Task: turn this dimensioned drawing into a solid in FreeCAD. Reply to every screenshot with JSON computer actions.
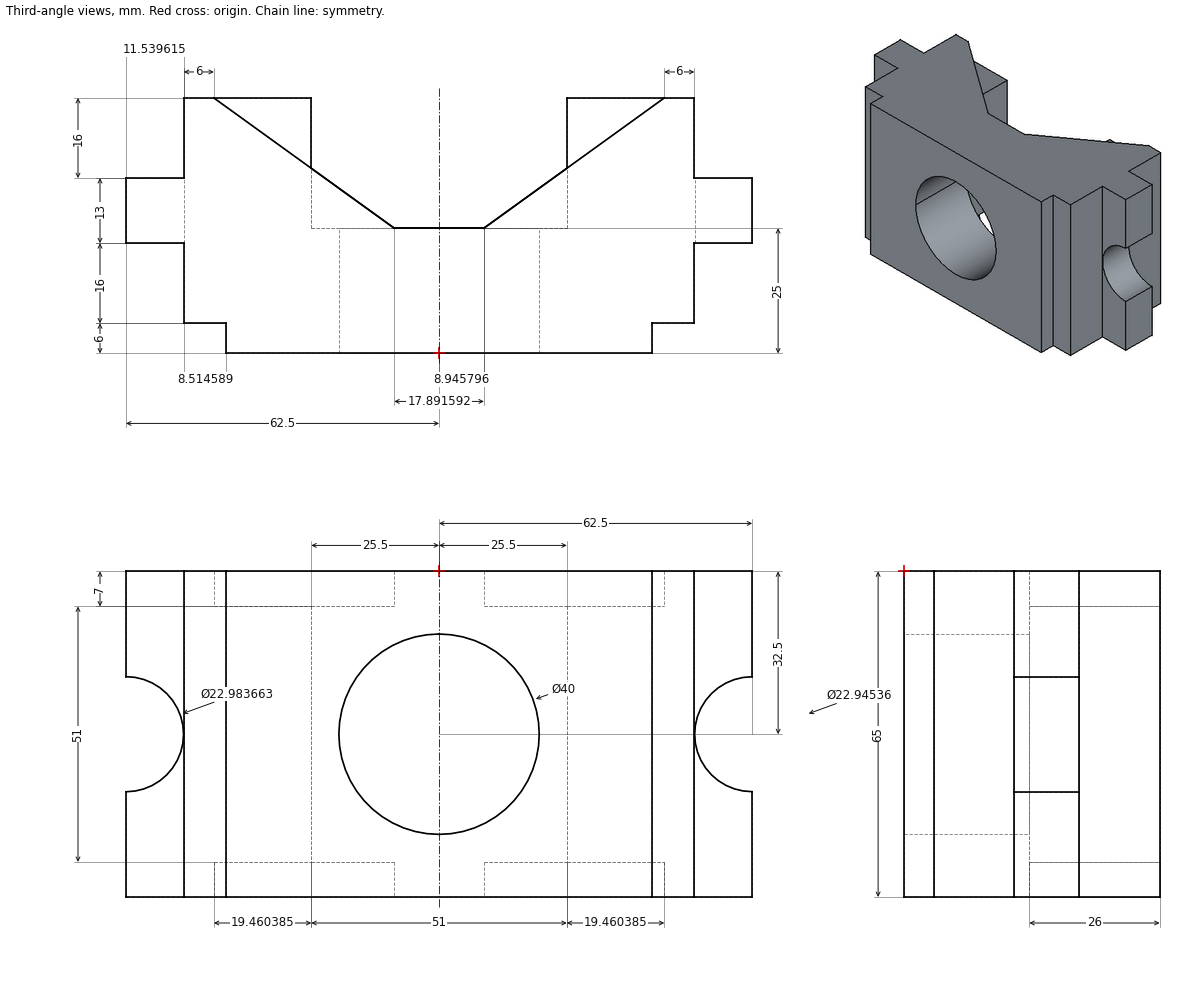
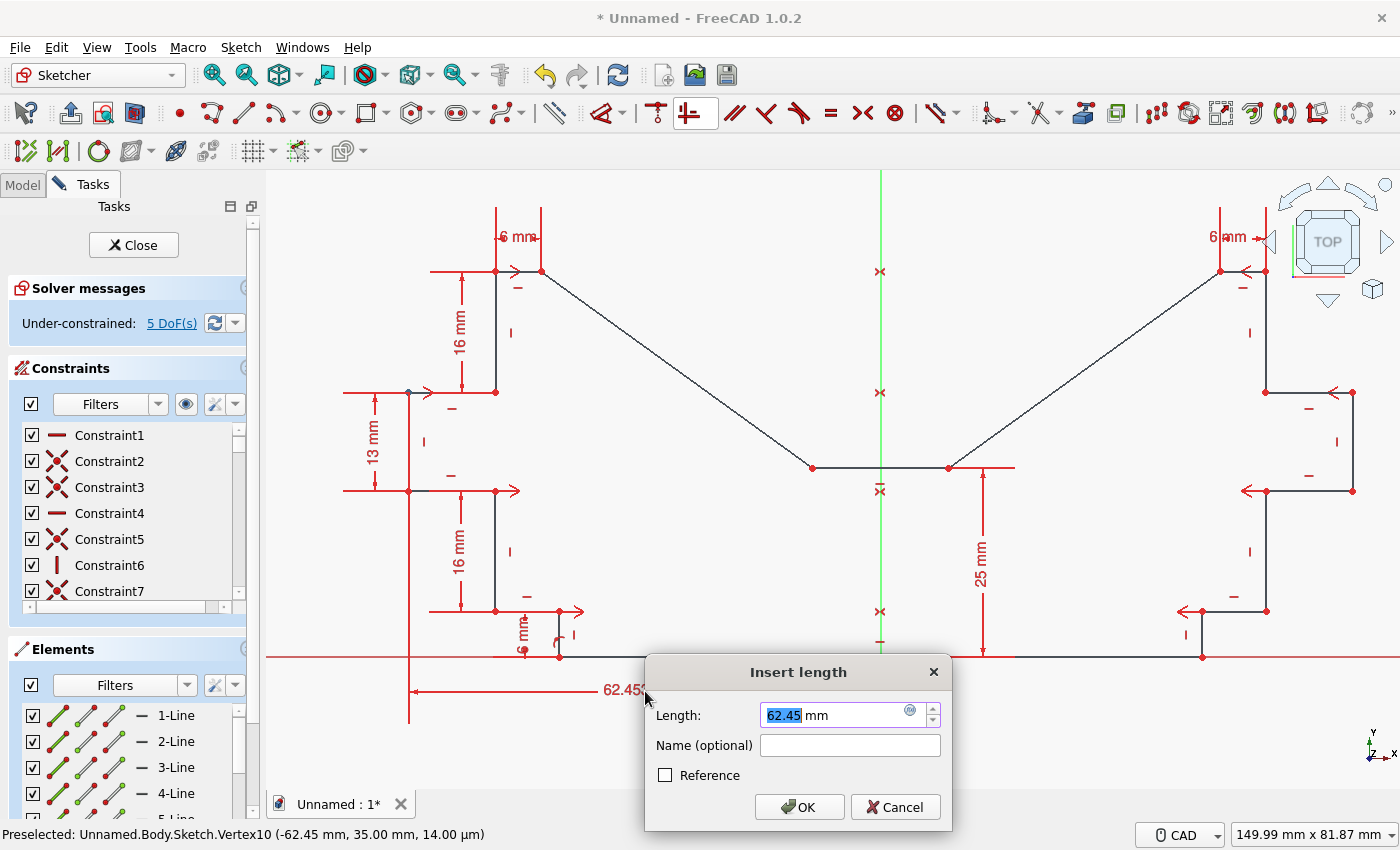
{"action": "type", "text": "62.5"}
{"action": "key", "text": "Return"}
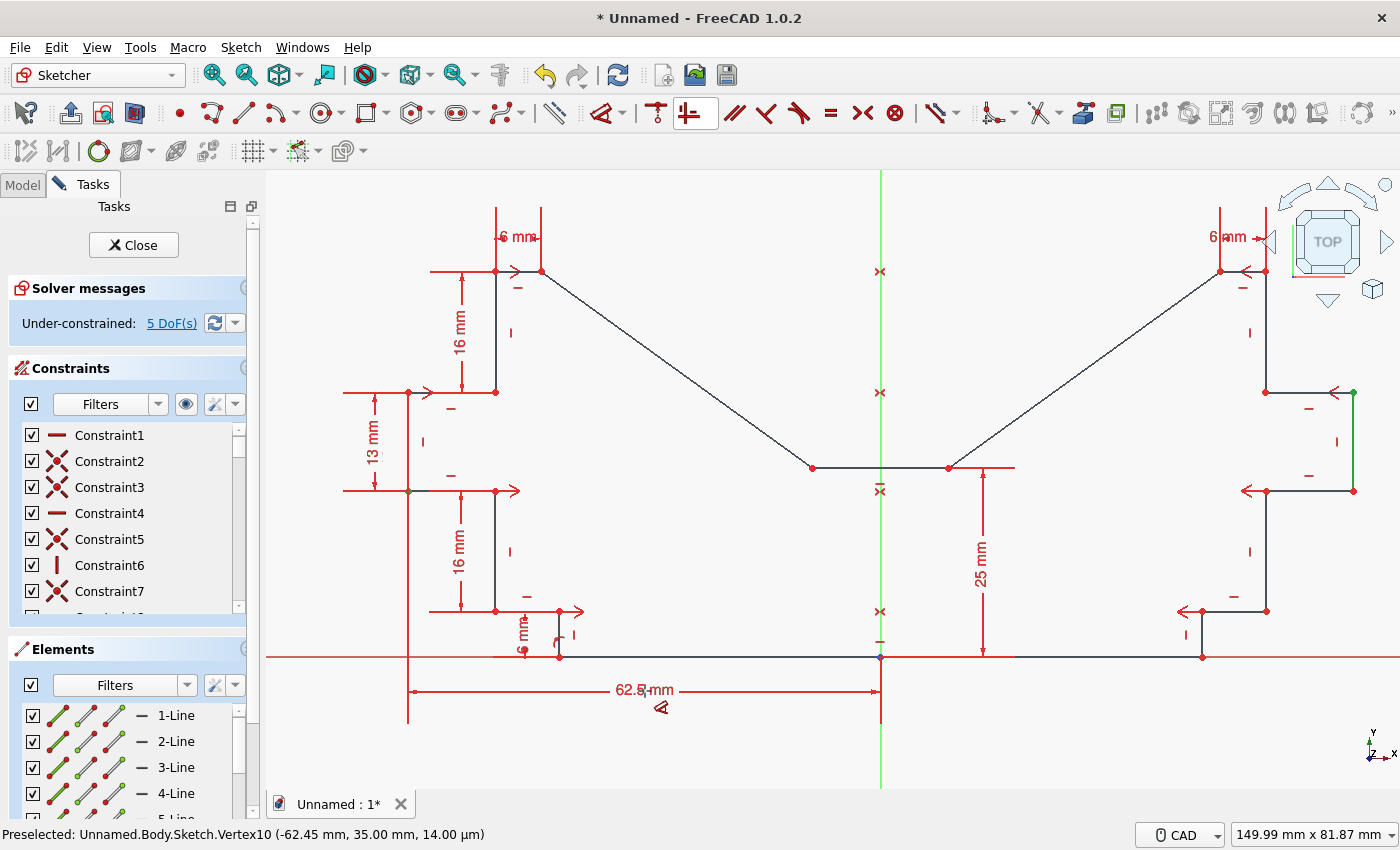
{"action": "left_click", "coordinate": [514, 612]}
{"action": "left_click", "coordinate": [527, 578]}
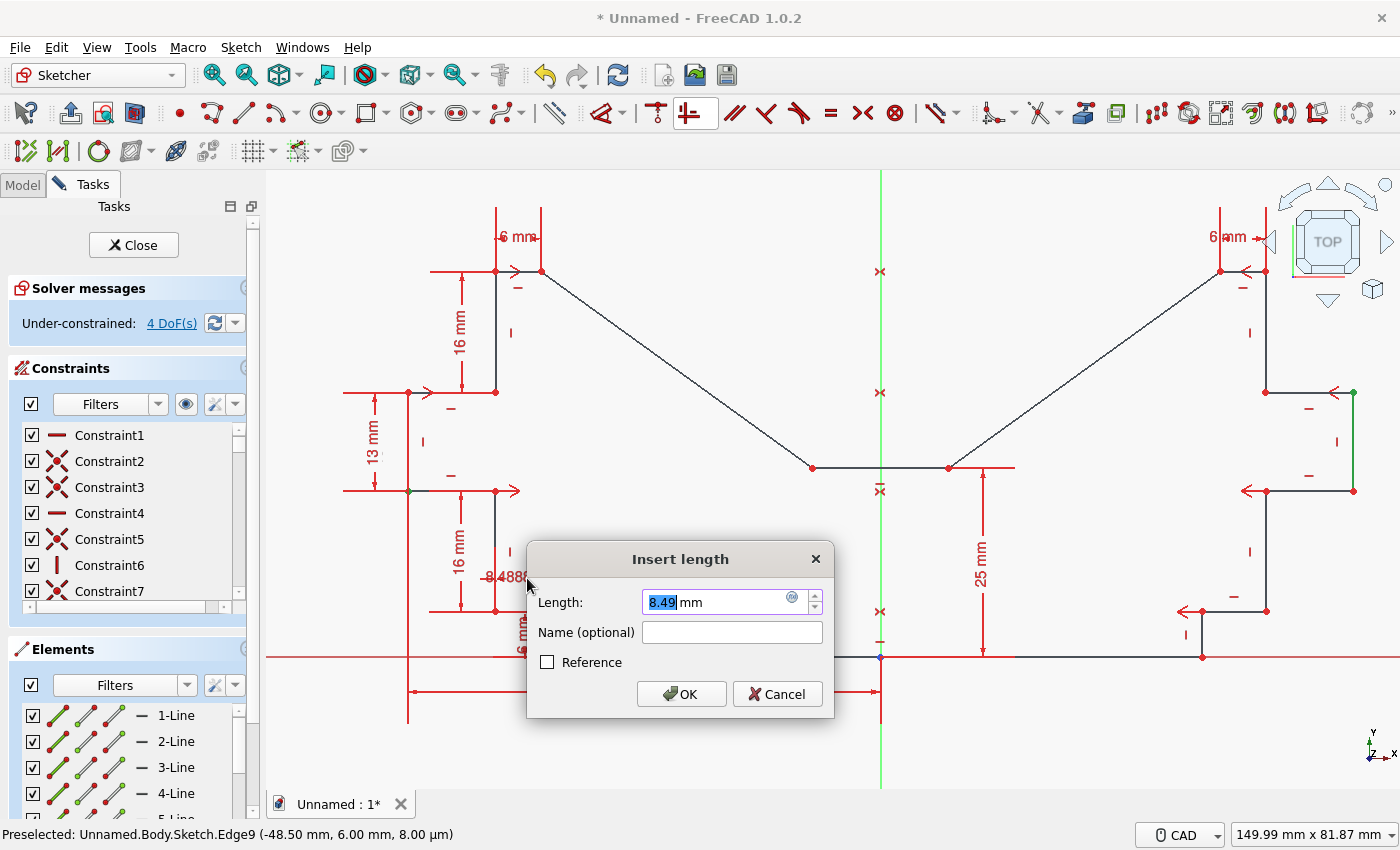
{"action": "type", "text": "8.514589"}
{"action": "key", "text": "Return"}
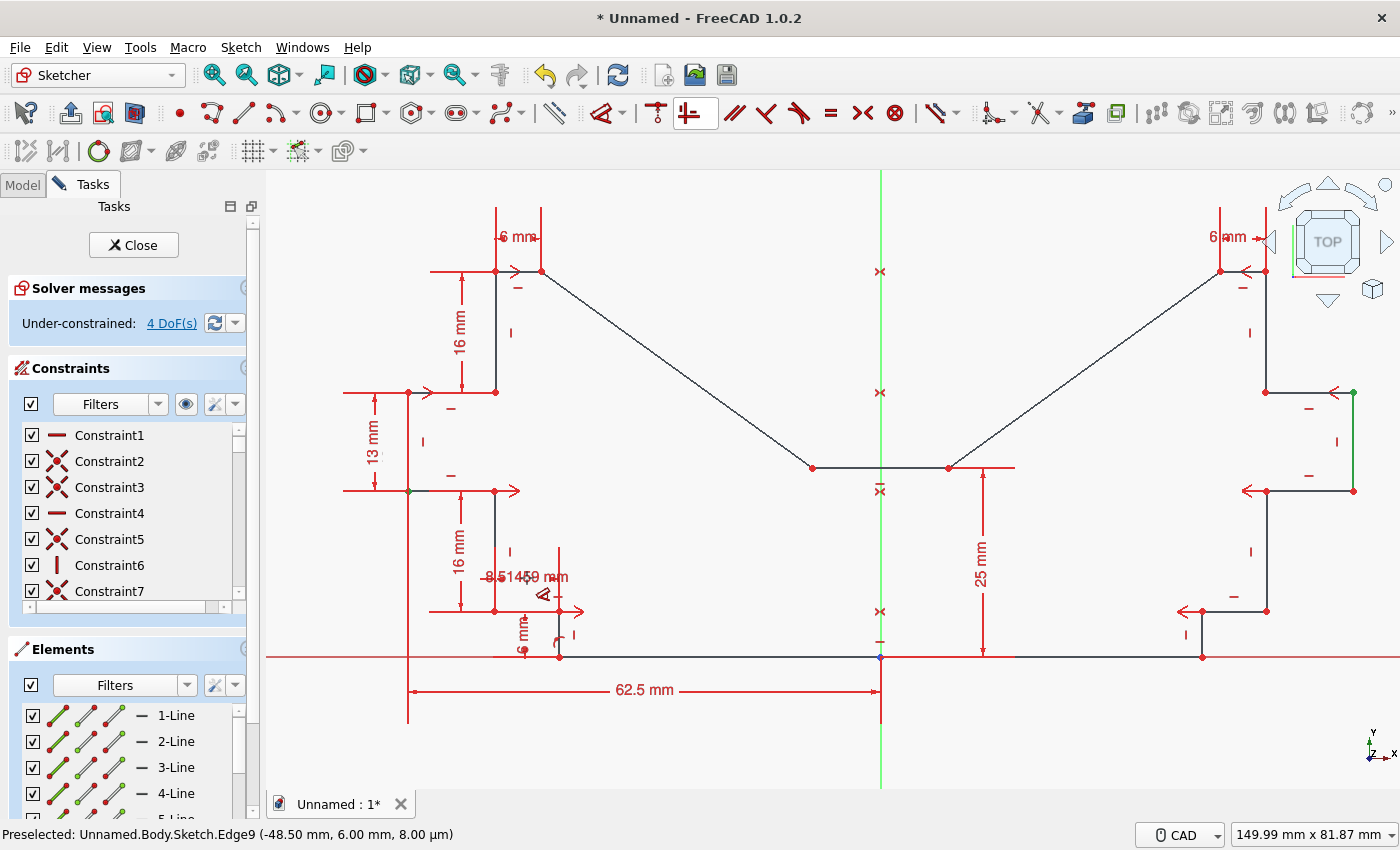
{"action": "left_click", "coordinate": [908, 468]}
{"action": "left_click", "coordinate": [849, 502]}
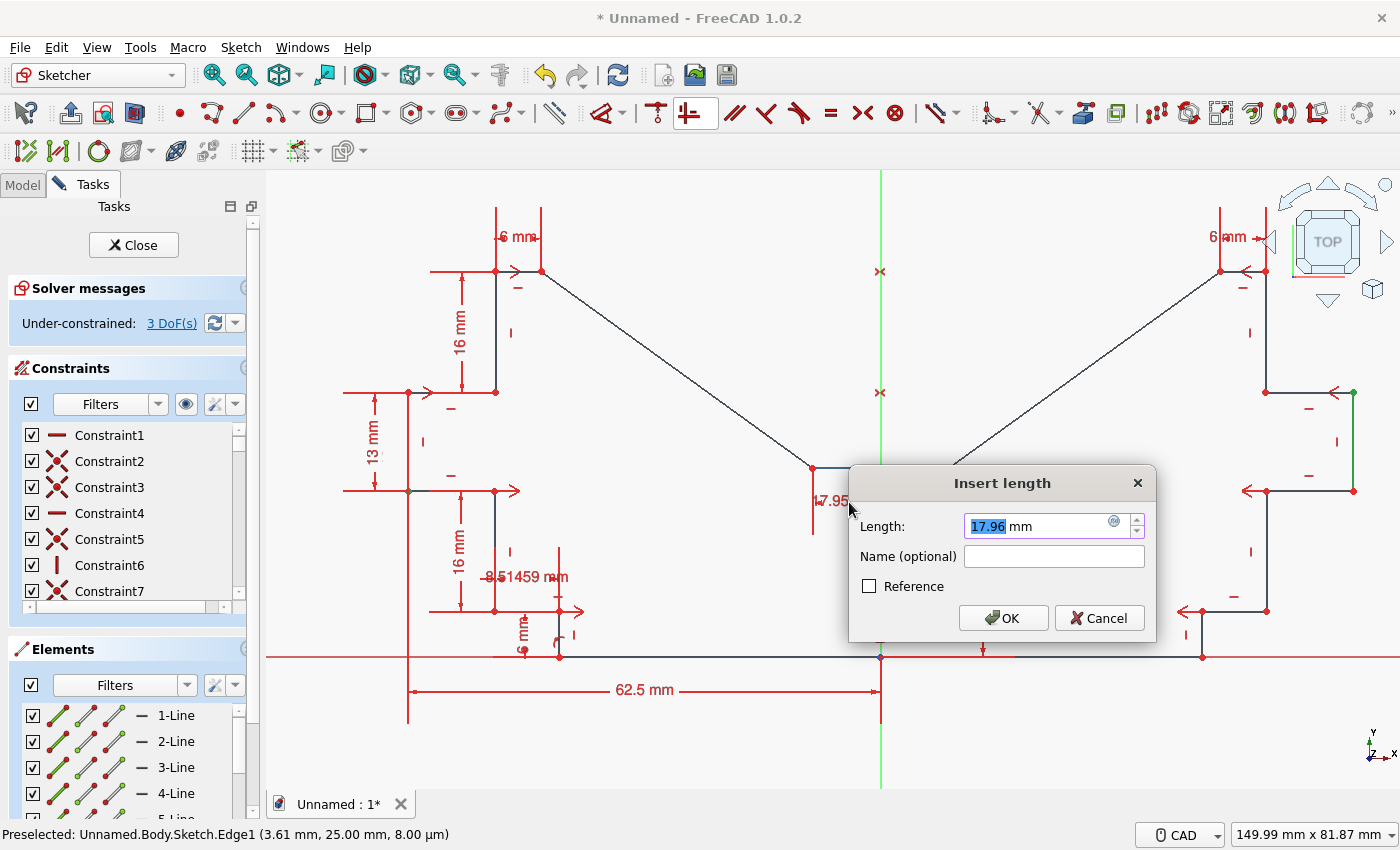
{"action": "type", "text": "17.891592"}
{"action": "key", "text": "Return"}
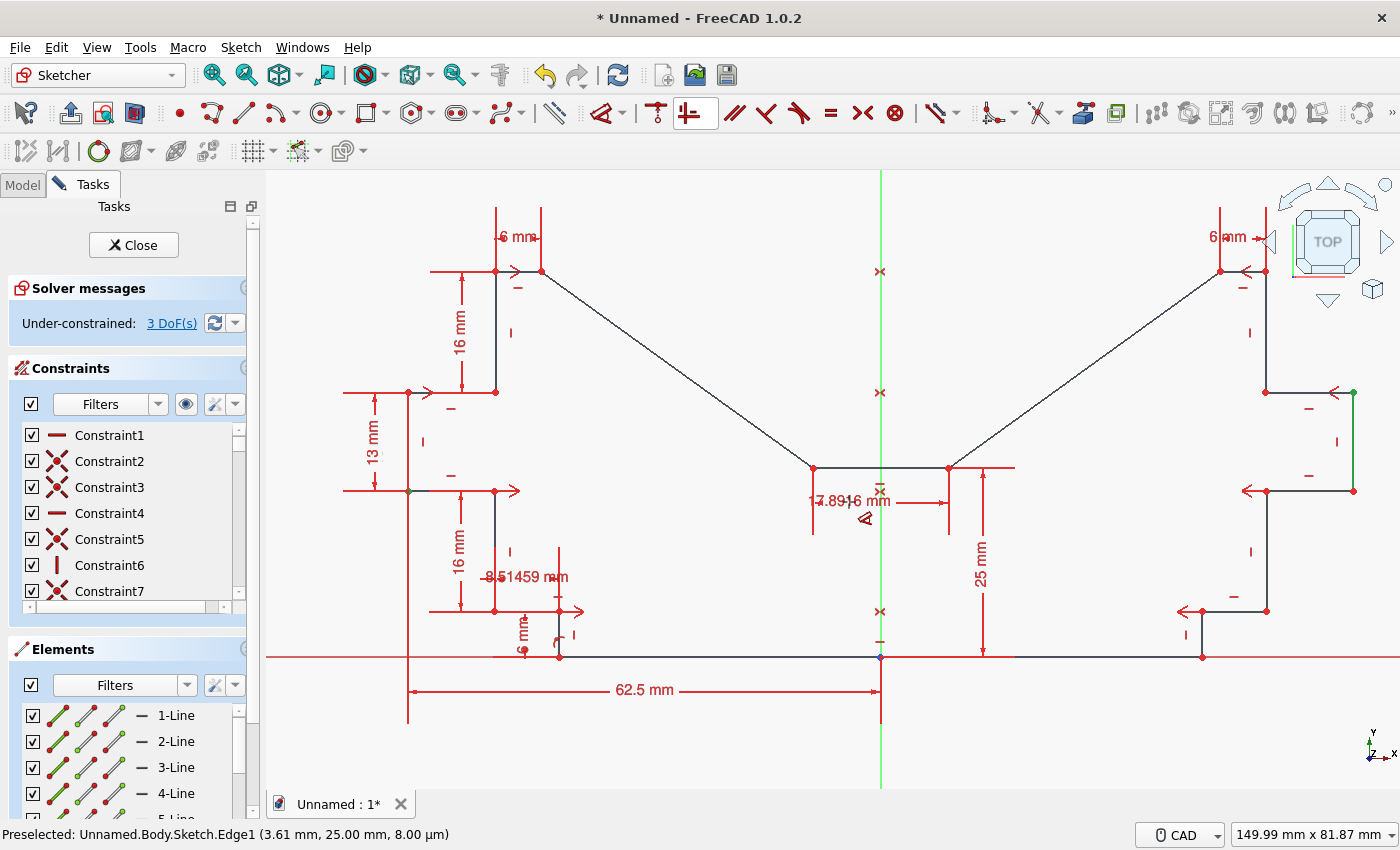
{"action": "left_click", "coordinate": [469, 393]}
{"action": "left_click", "coordinate": [452, 359]}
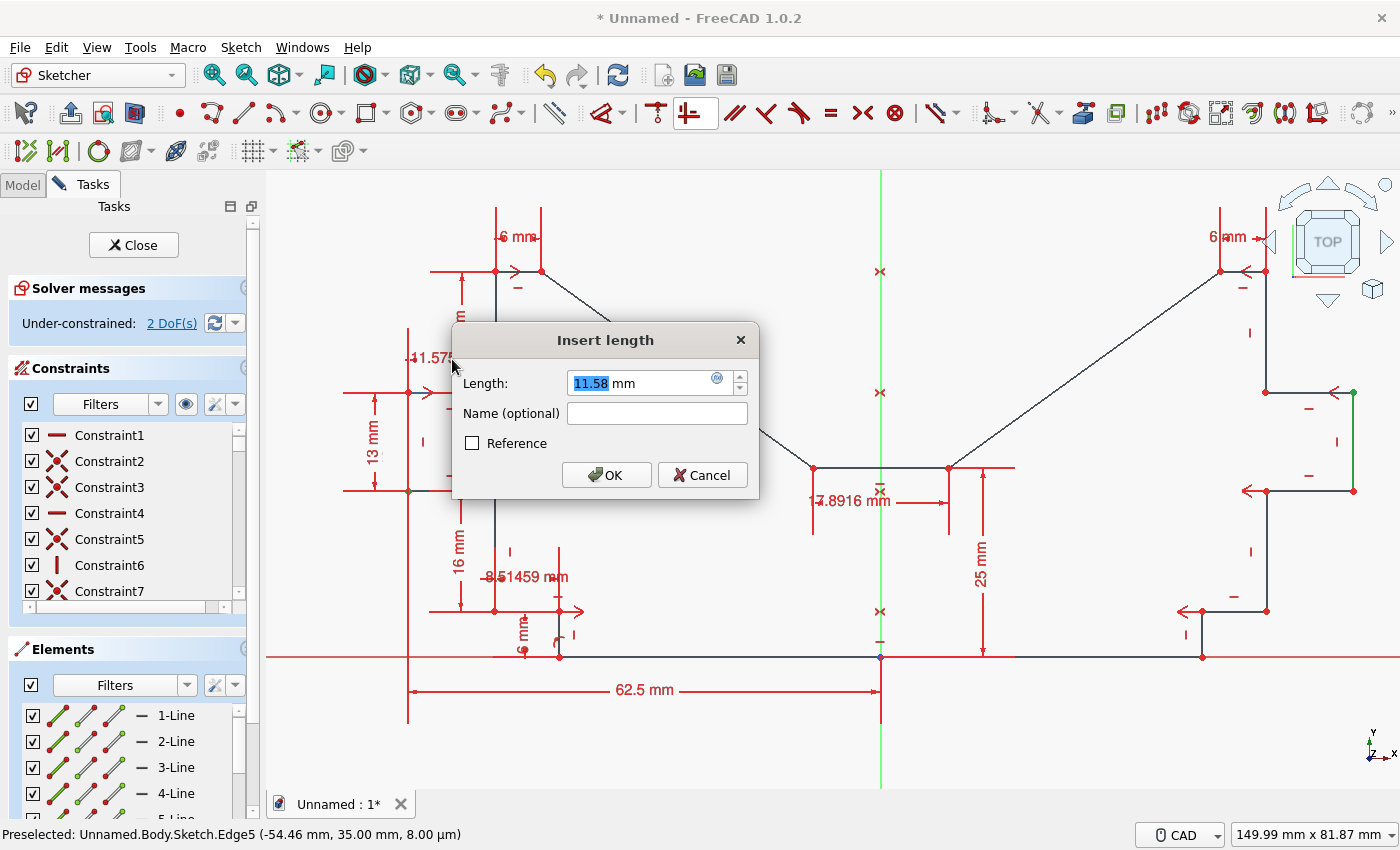
{"action": "type", "text": "11.539615"}
{"action": "key", "text": "Return"}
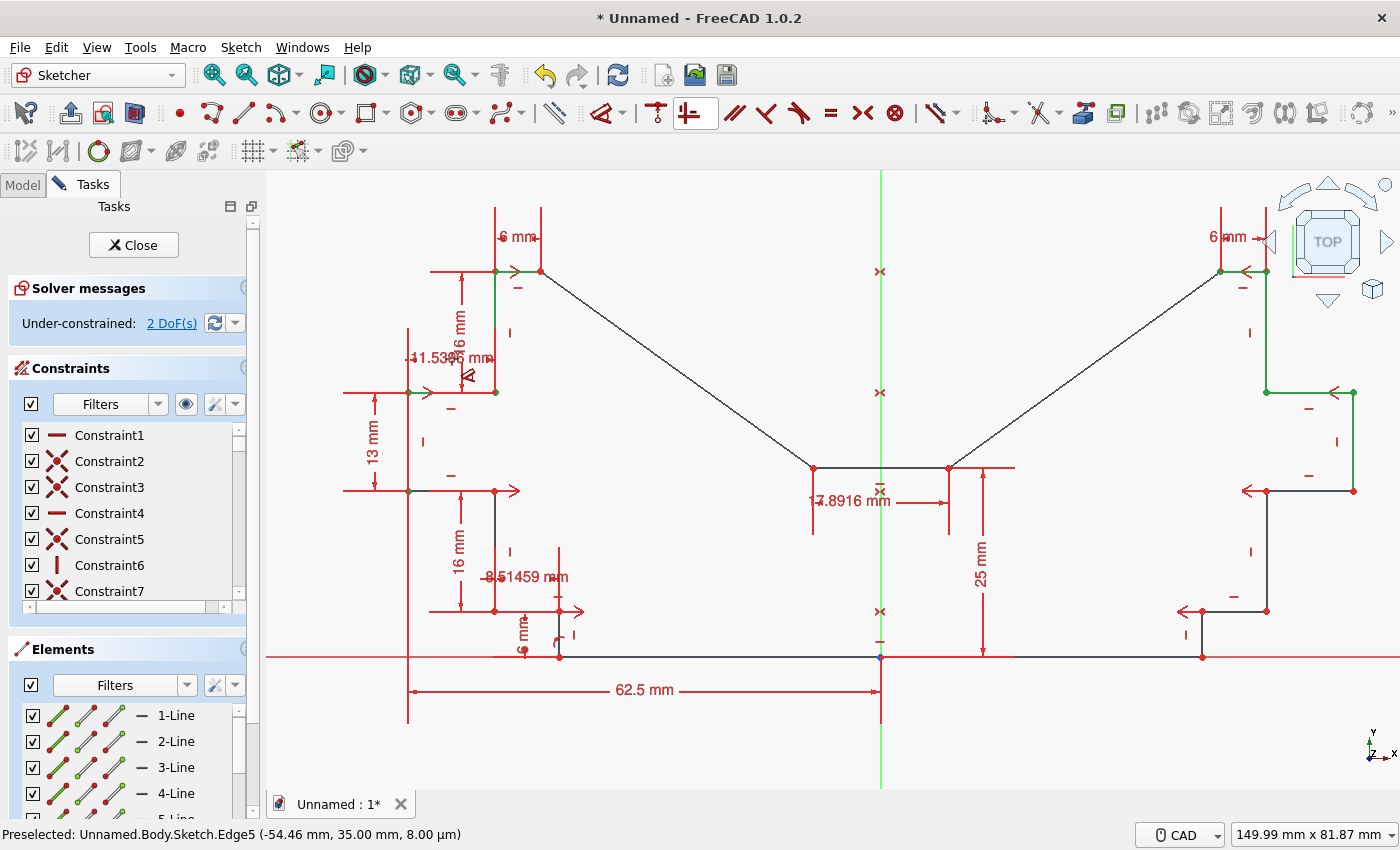
{"action": "left_click", "coordinate": [434, 491]}
{"action": "left_click", "coordinate": [452, 525]}